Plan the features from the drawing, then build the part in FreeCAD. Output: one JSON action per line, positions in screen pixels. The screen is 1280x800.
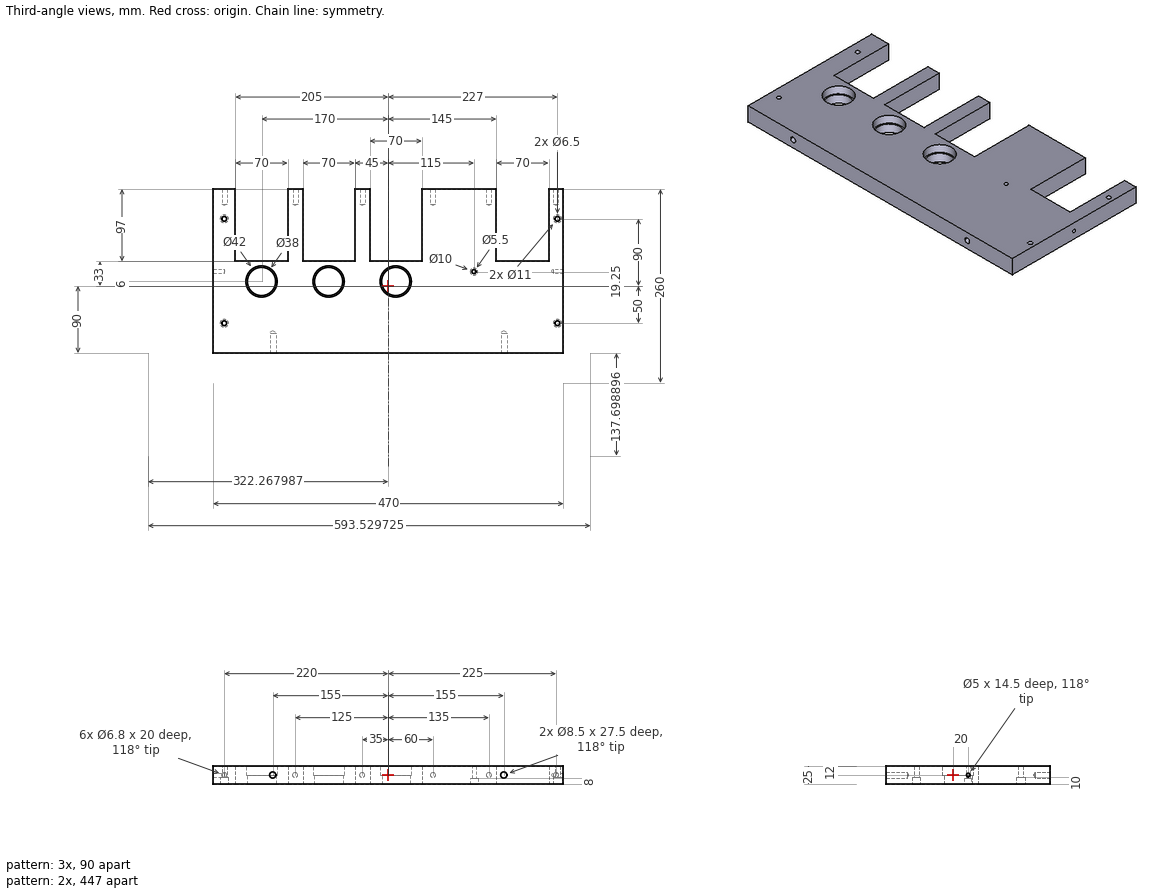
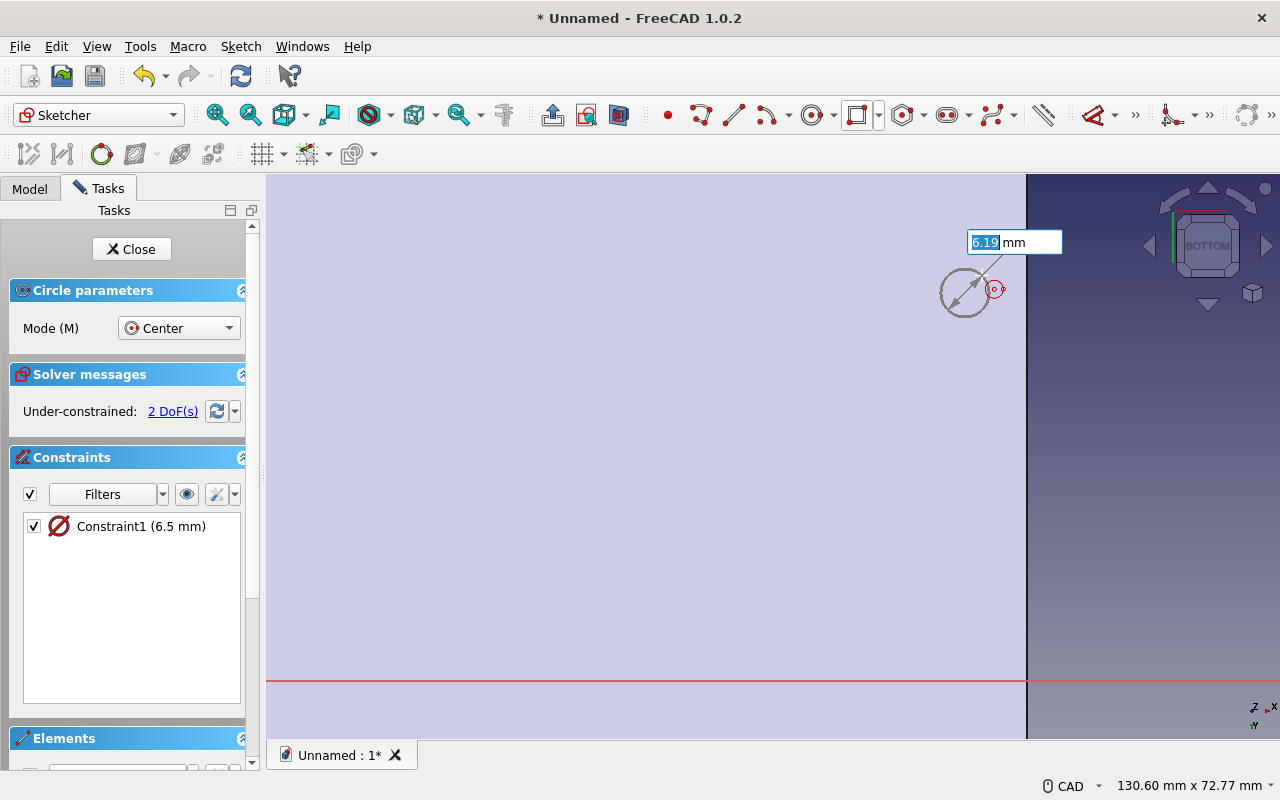
{"action": "type", "text": "6.5"}
{"action": "key", "text": "Return"}
{"action": "key", "text": "Escape"}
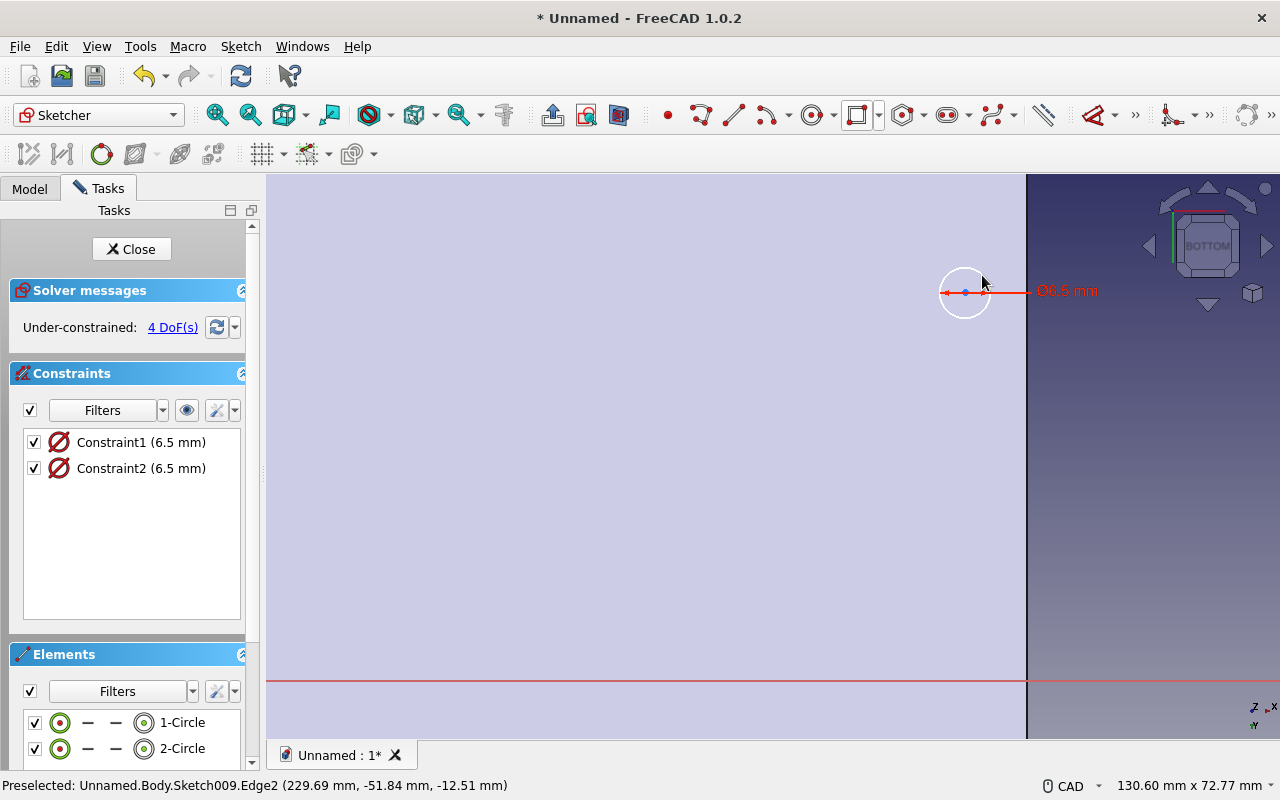
{"action": "left_click", "coordinate": [1092, 116]}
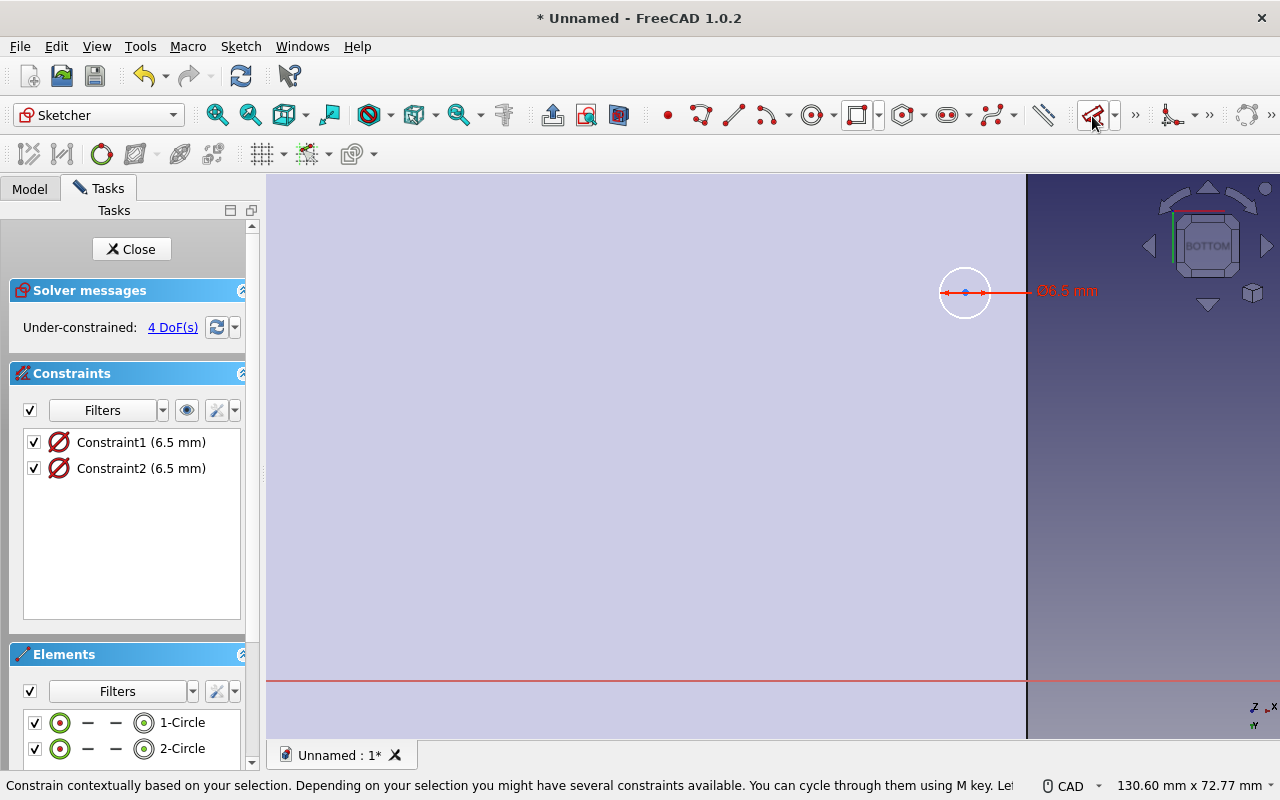
{"action": "scroll", "coordinate": [967, 293], "scroll_direction": "down", "scroll_amount": 6}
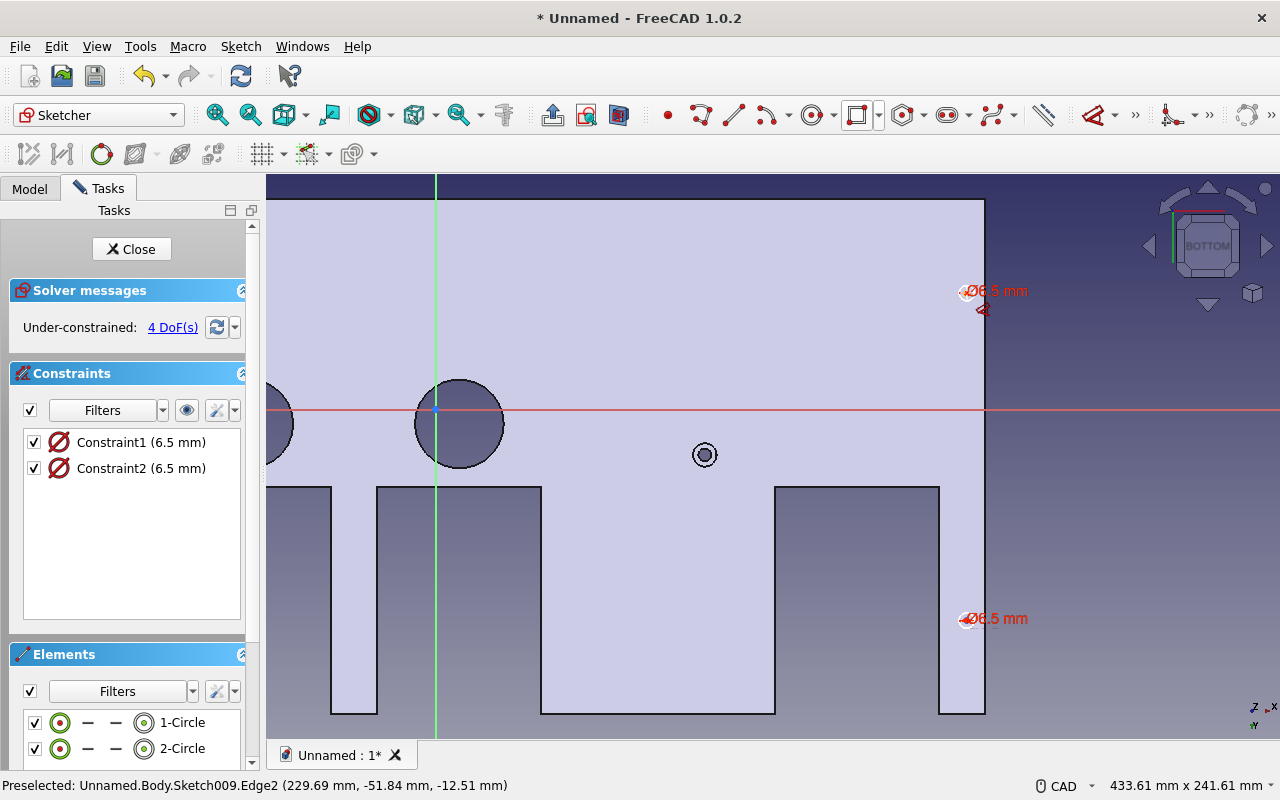
{"action": "left_click", "coordinate": [967, 621]}
{"action": "left_click", "coordinate": [402, 515]}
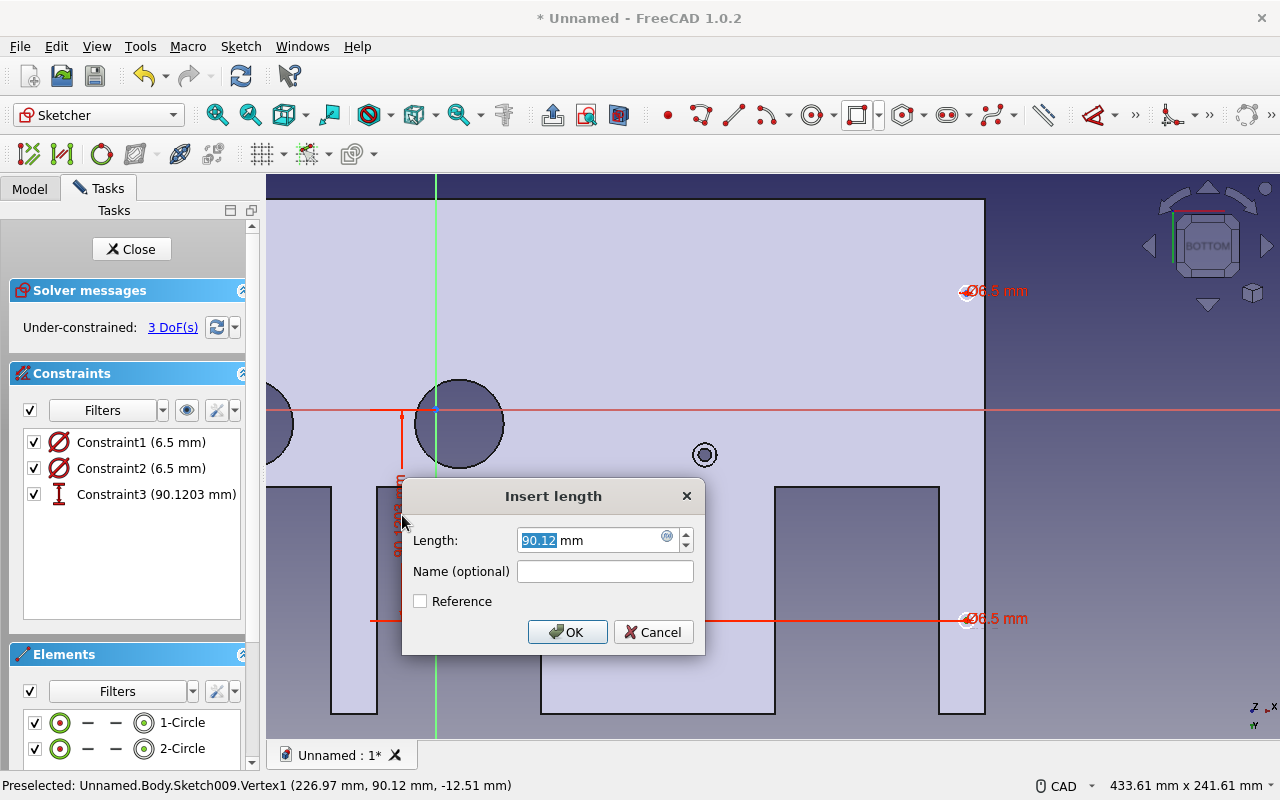
{"action": "type", "text": "90"}
{"action": "key", "text": "Return"}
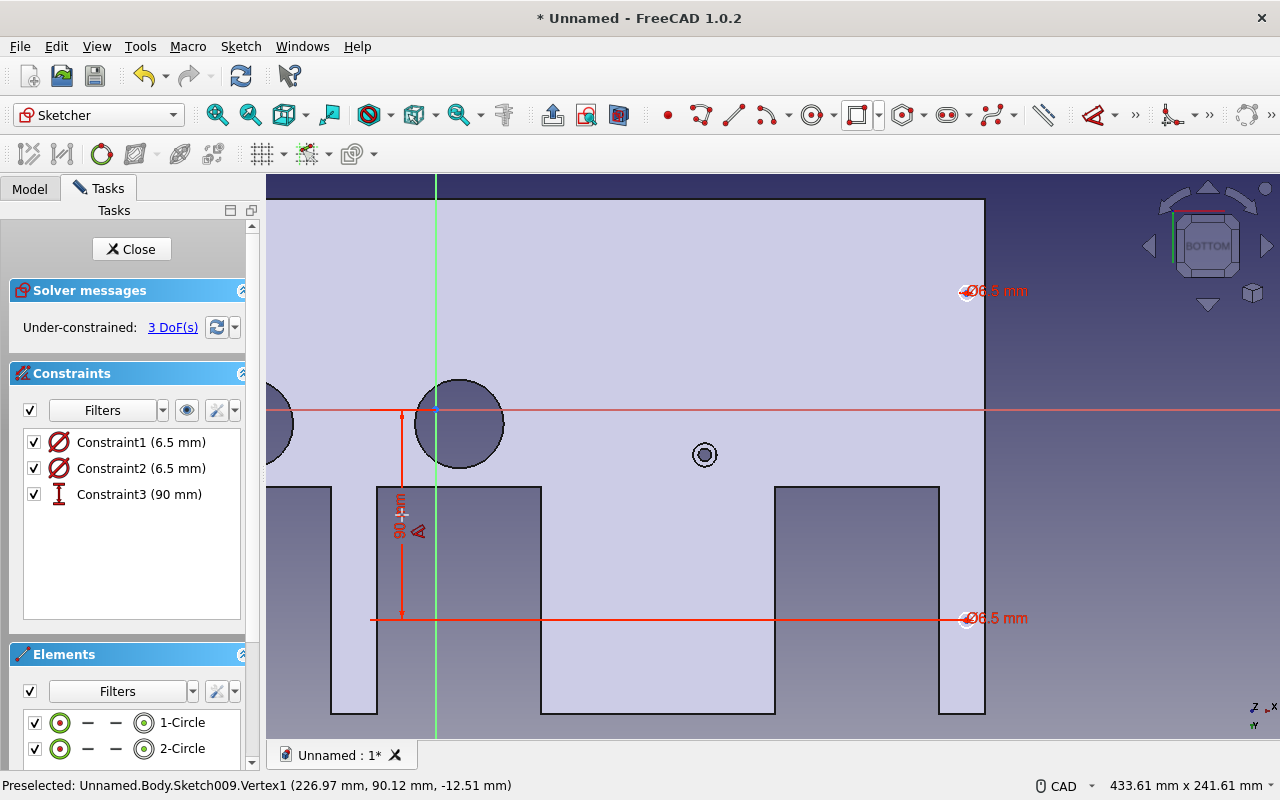
{"action": "left_click", "coordinate": [967, 293]}
{"action": "left_click", "coordinate": [402, 352]}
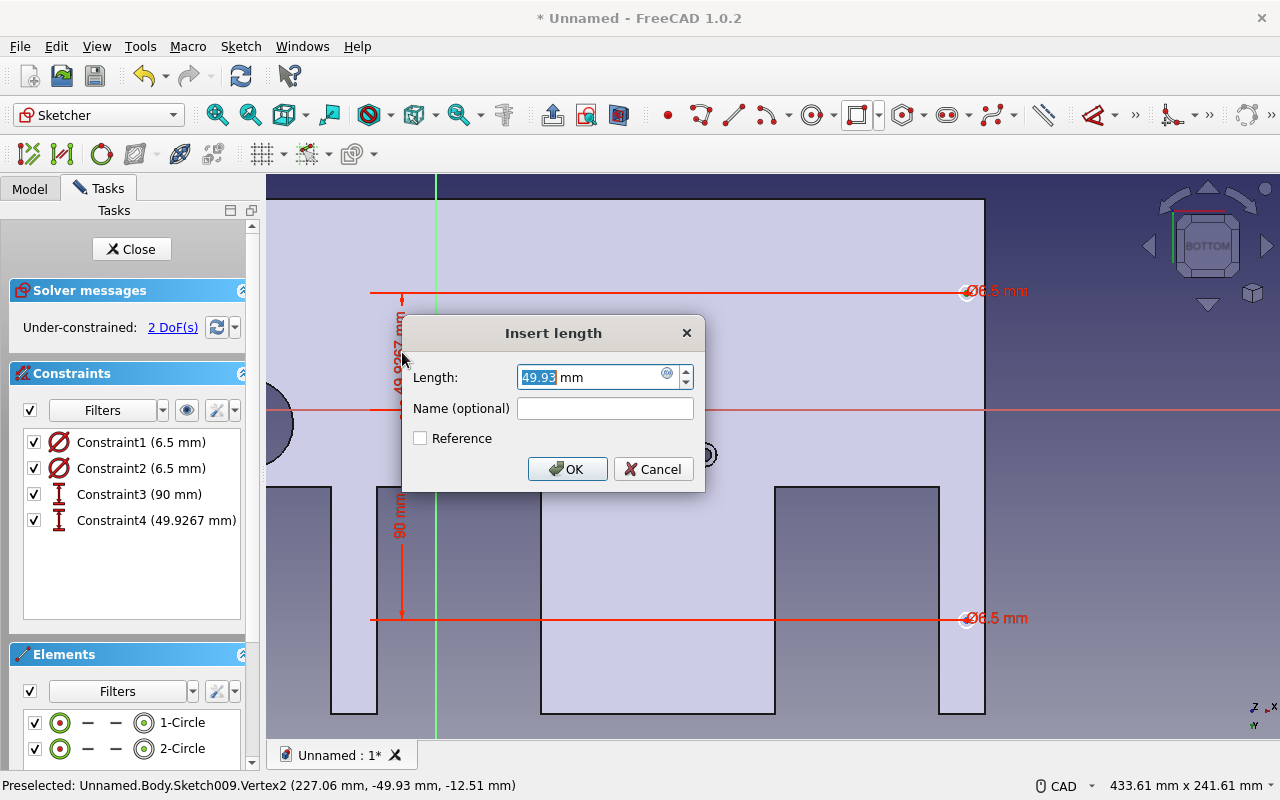
{"action": "type", "text": "50"}
{"action": "key", "text": "Return"}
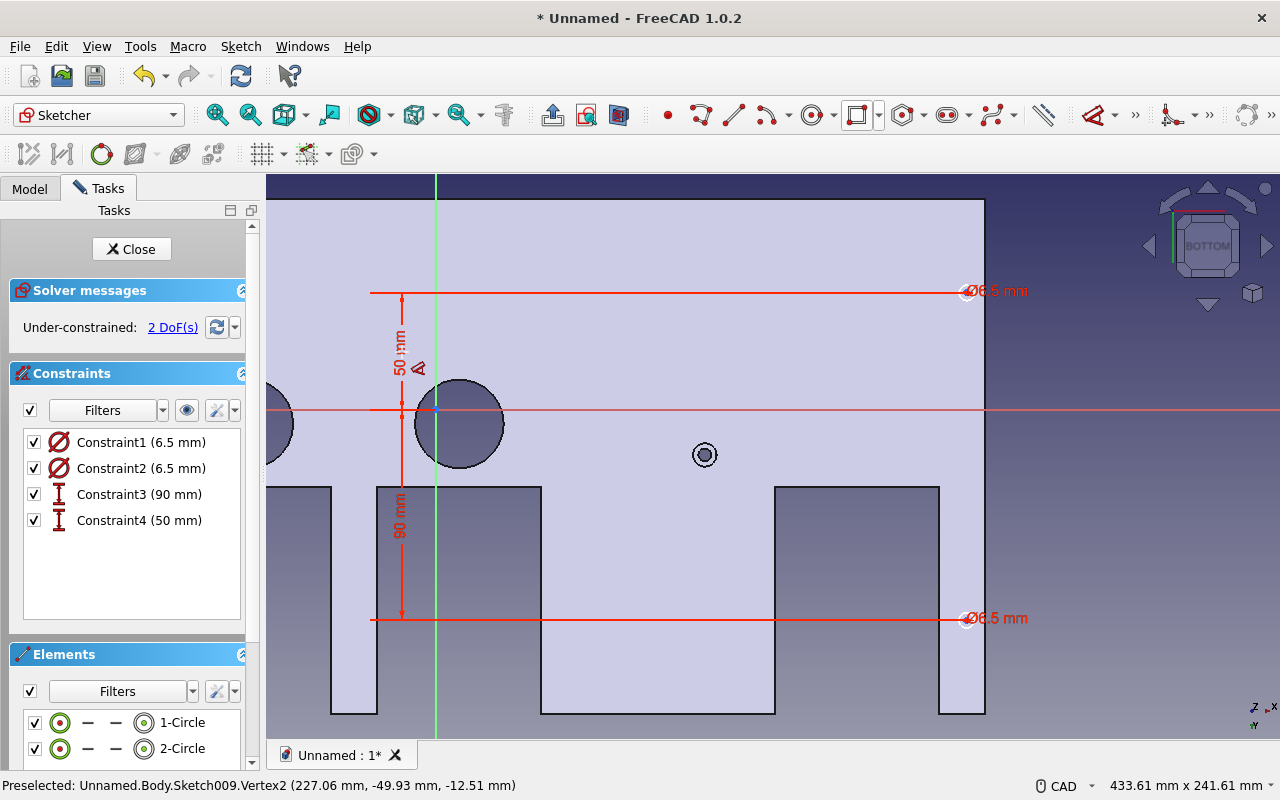
{"action": "left_click", "coordinate": [967, 620]}
{"action": "left_click", "coordinate": [701, 654]}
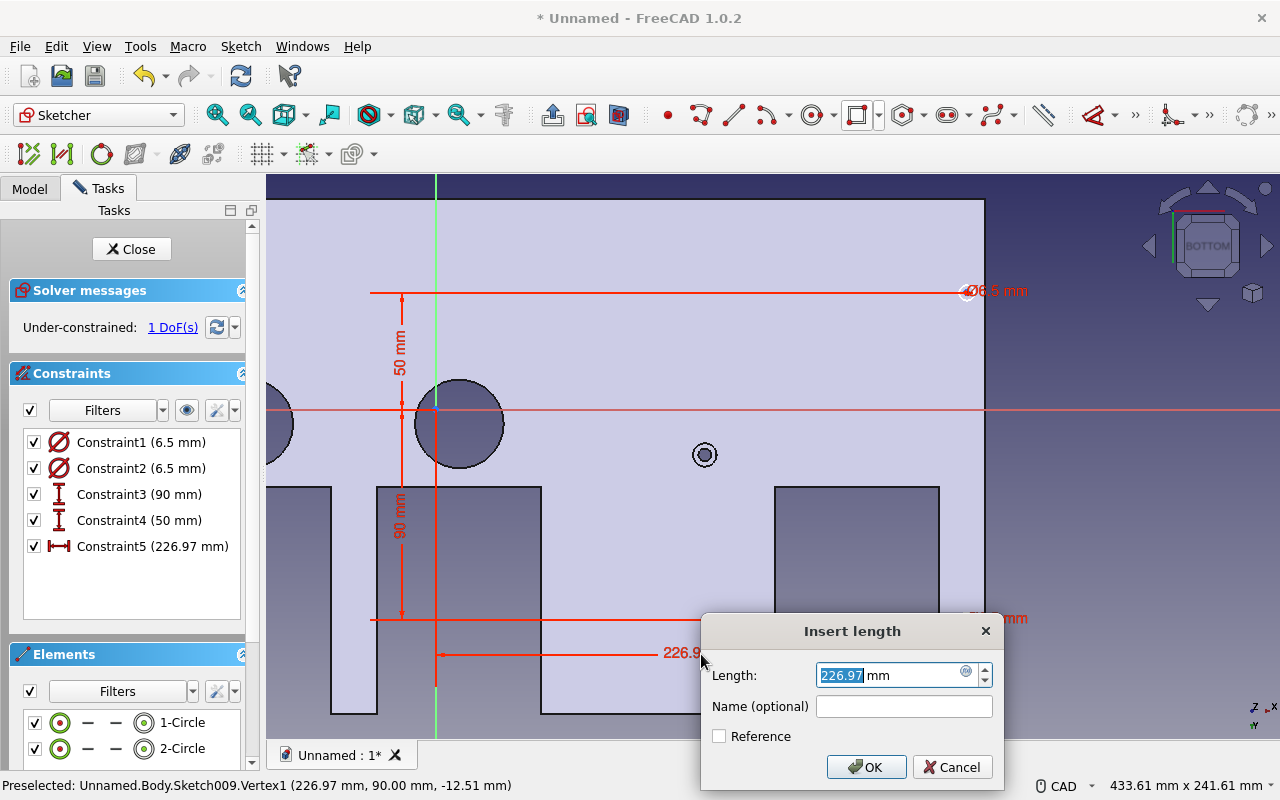
{"action": "type", "text": "227"}
{"action": "key", "text": "Return"}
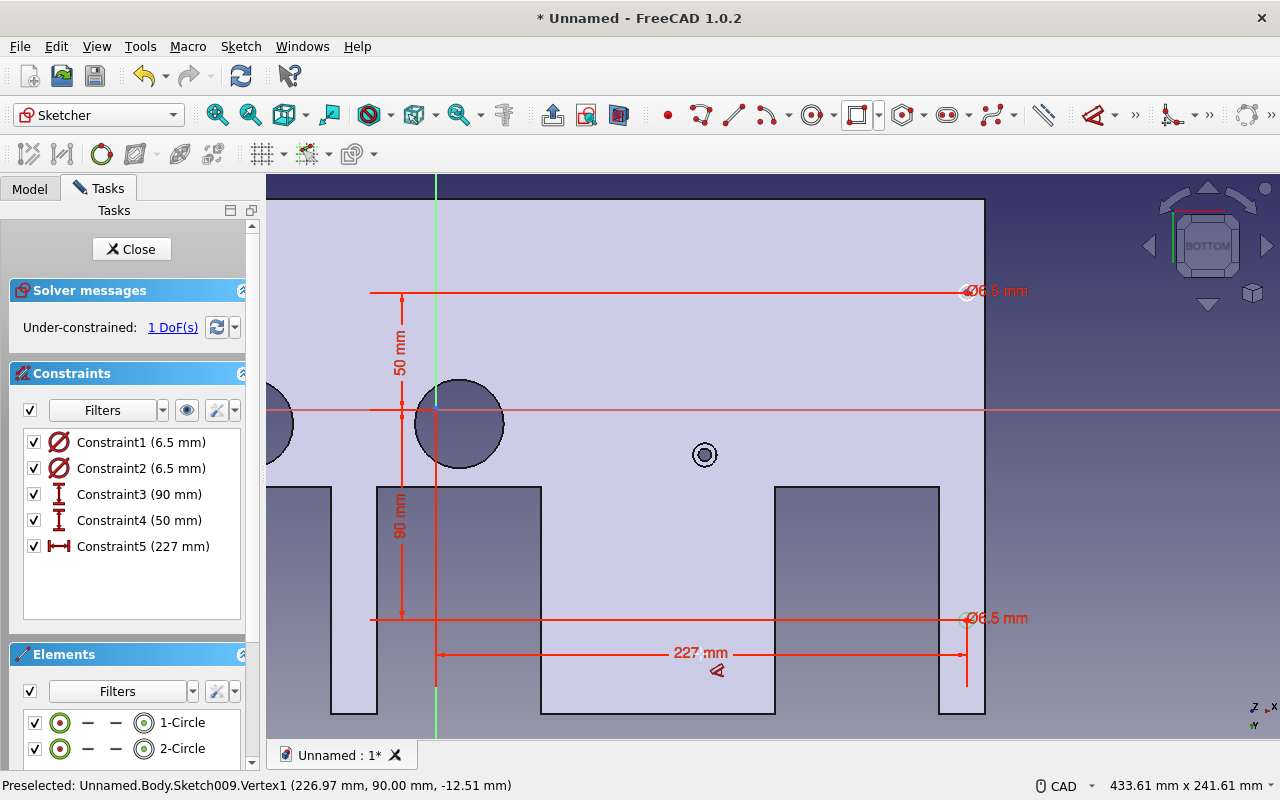
{"action": "left_click", "coordinate": [967, 293]}
{"action": "left_click", "coordinate": [701, 259]}